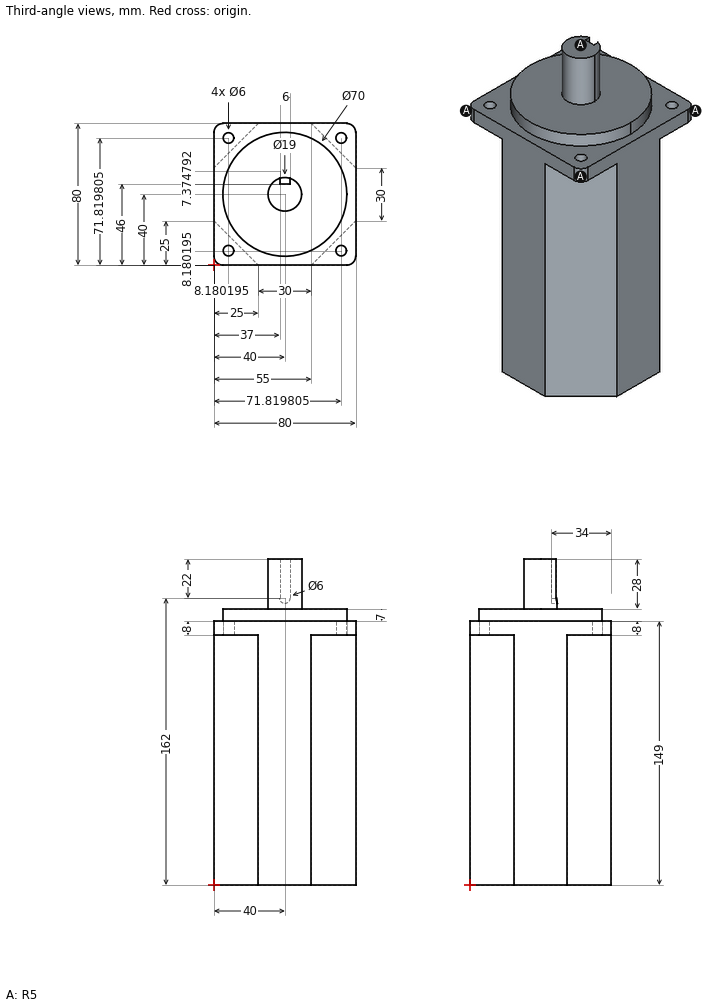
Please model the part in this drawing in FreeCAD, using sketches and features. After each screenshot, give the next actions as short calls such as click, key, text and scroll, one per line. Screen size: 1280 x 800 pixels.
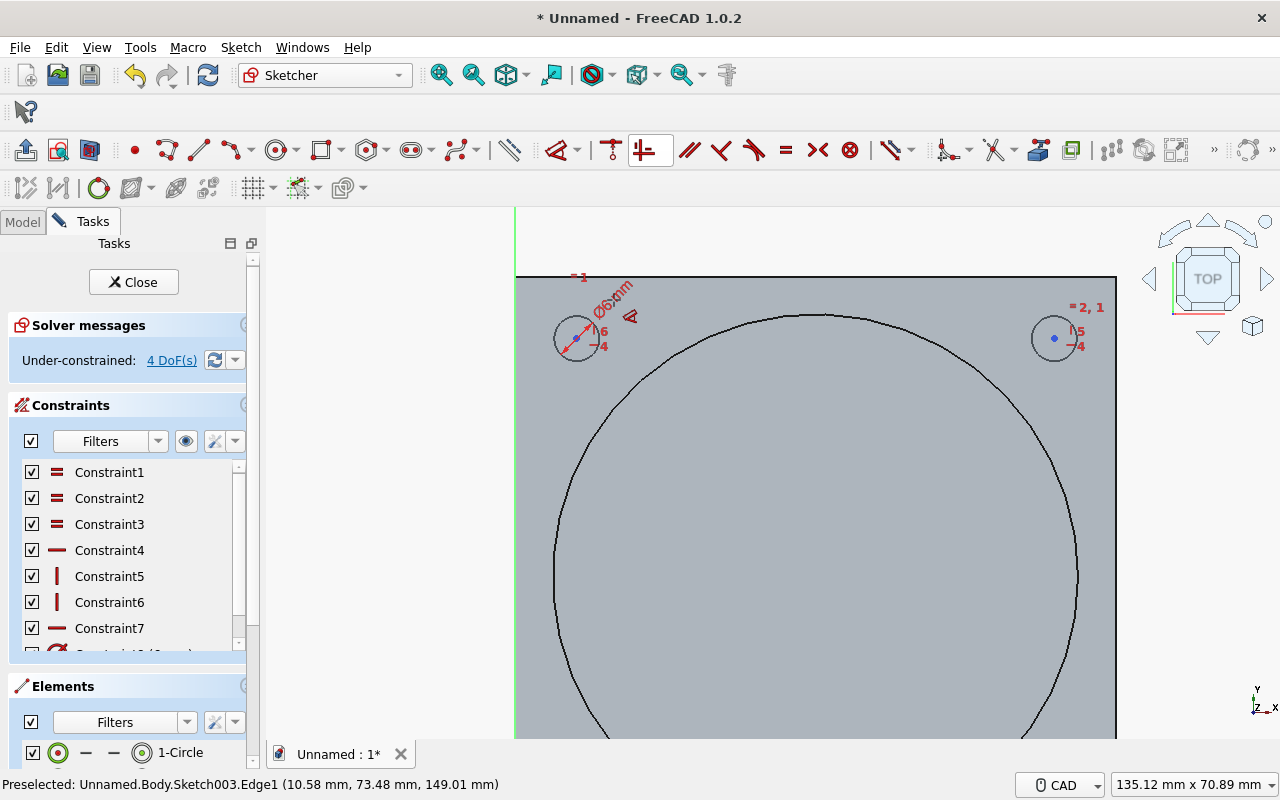
click(577, 339)
click(532, 305)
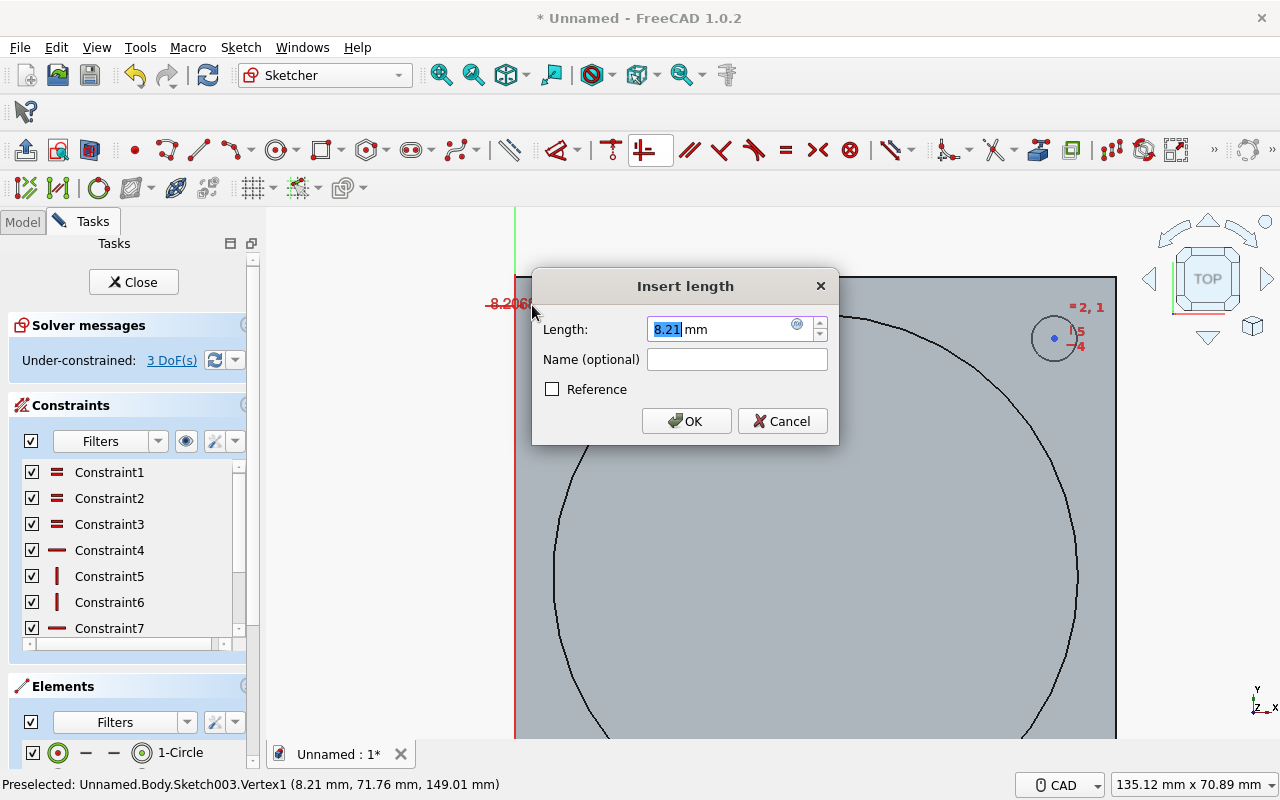
text(8.180195)
key(Return)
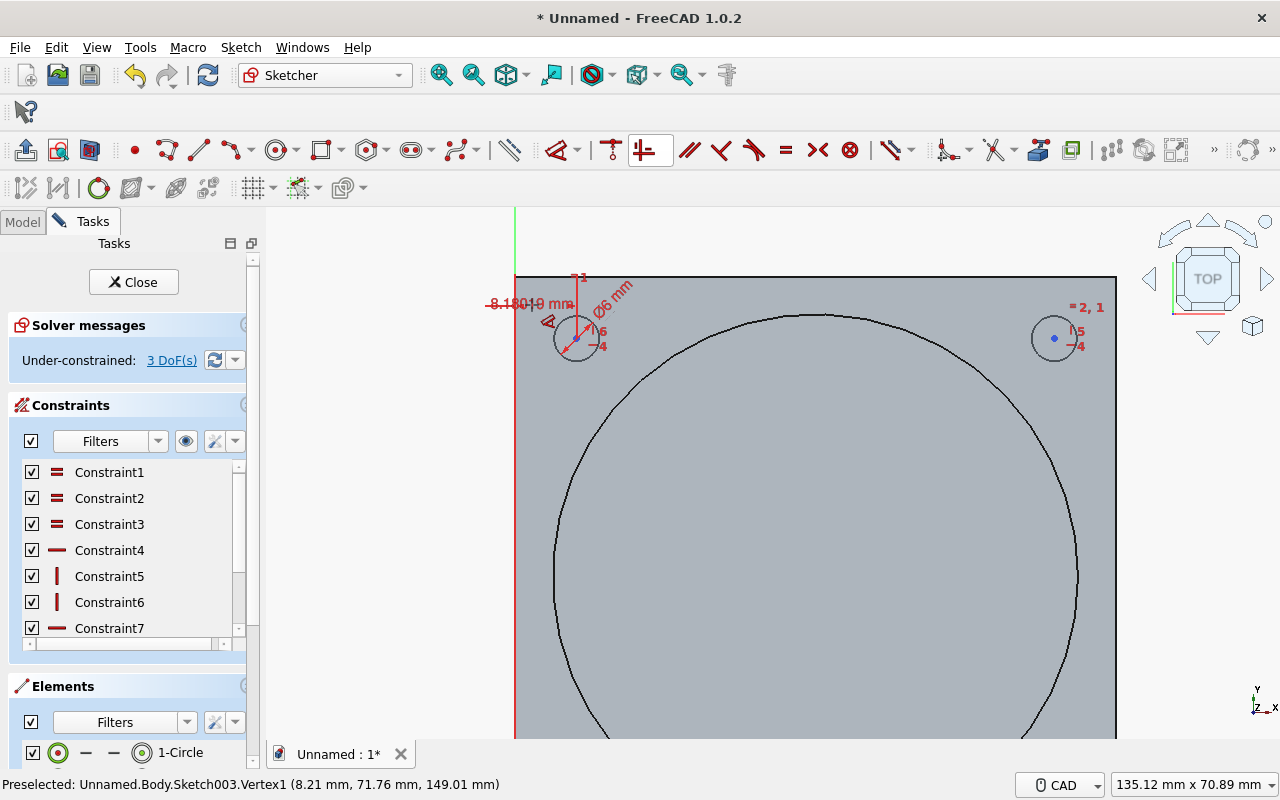
scroll(593, 323, down, 3)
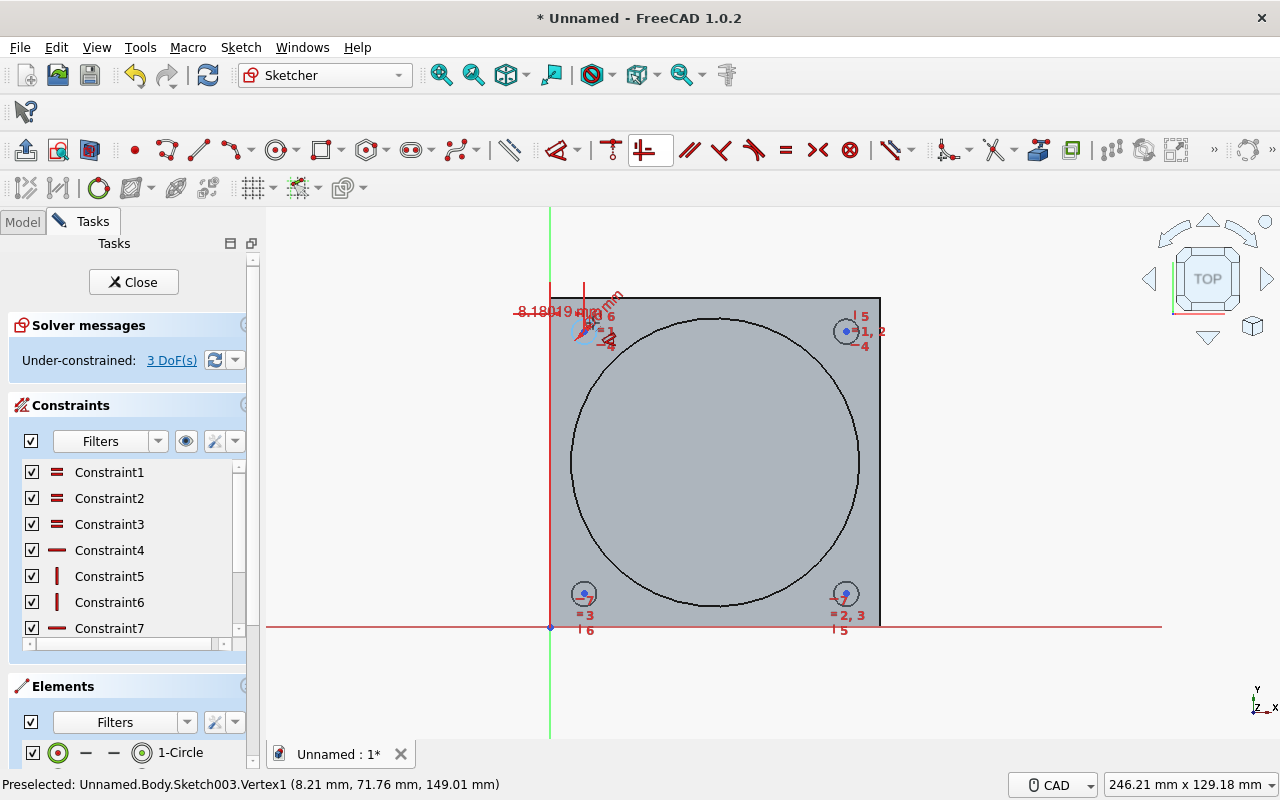
click(846, 594)
click(516, 611)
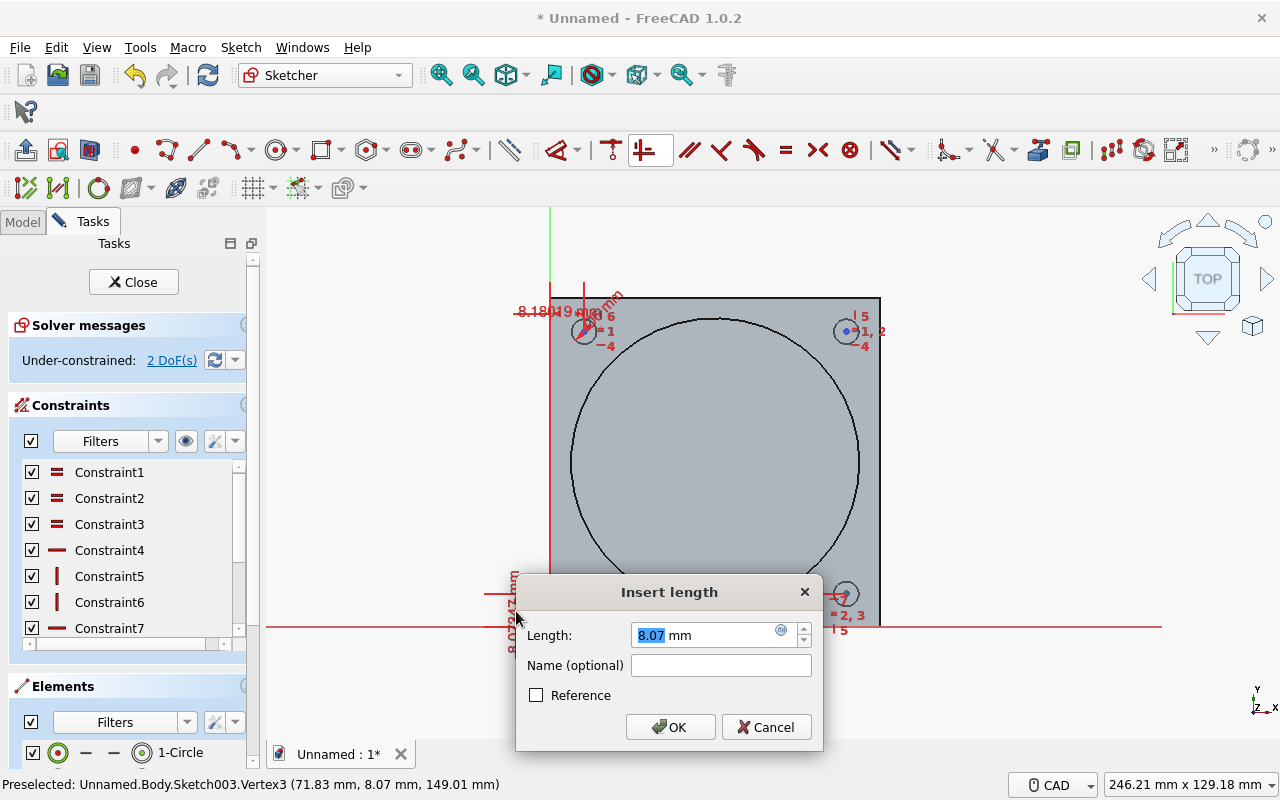
text(8.180195)
key(Return)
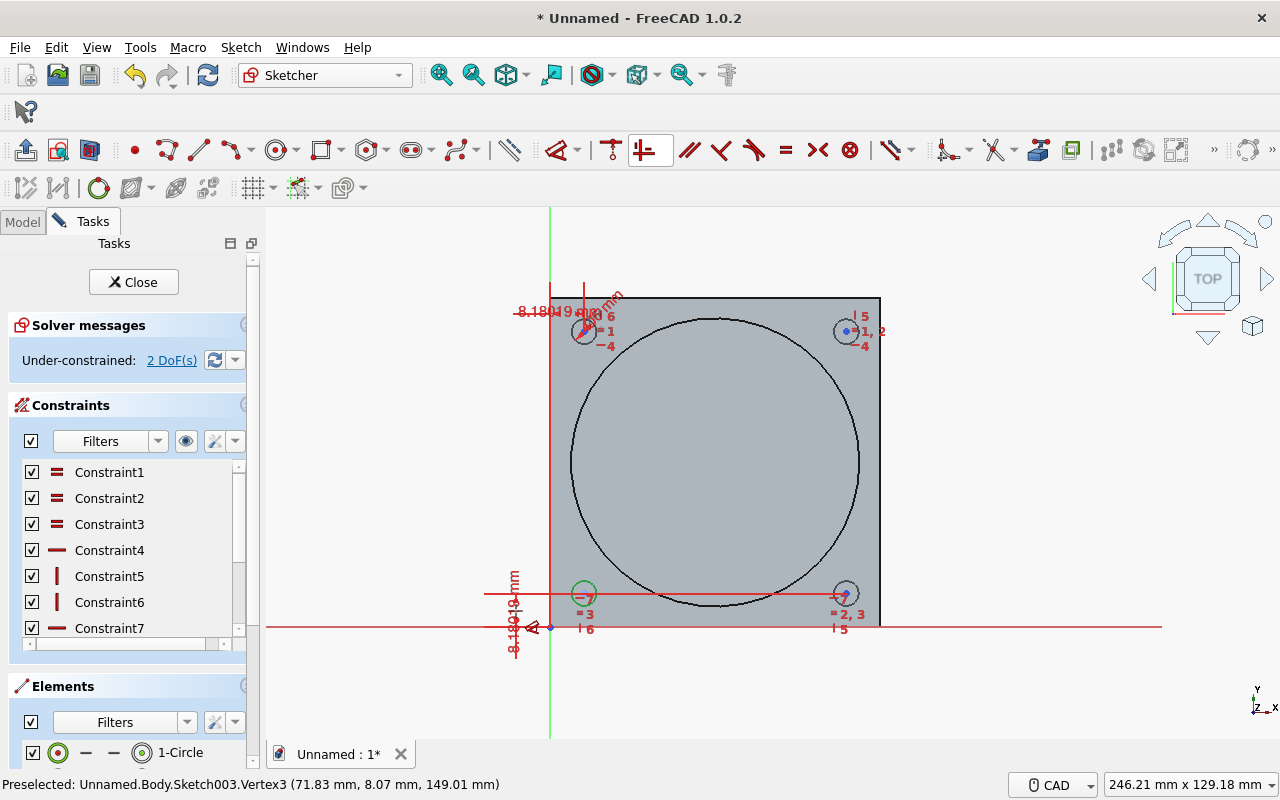
click(584, 332)
click(516, 479)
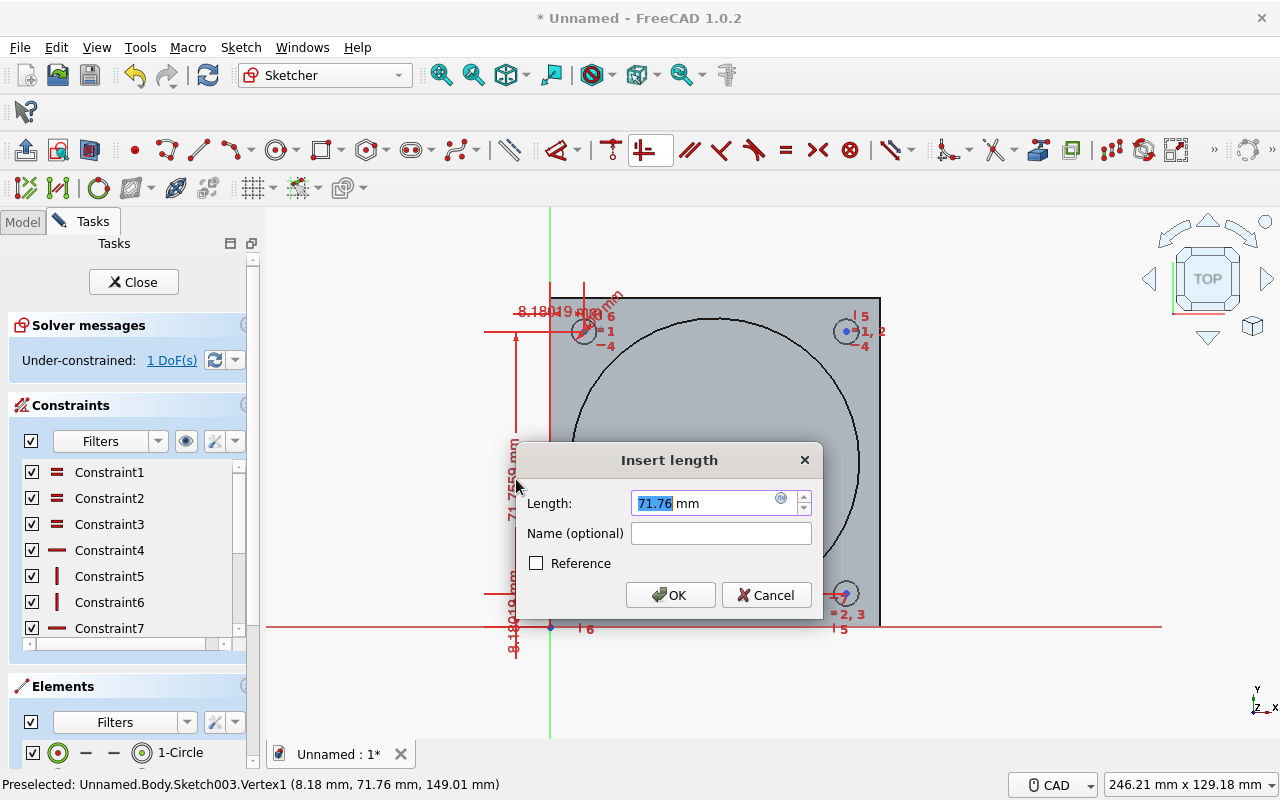
text(71.819805)
key(Return)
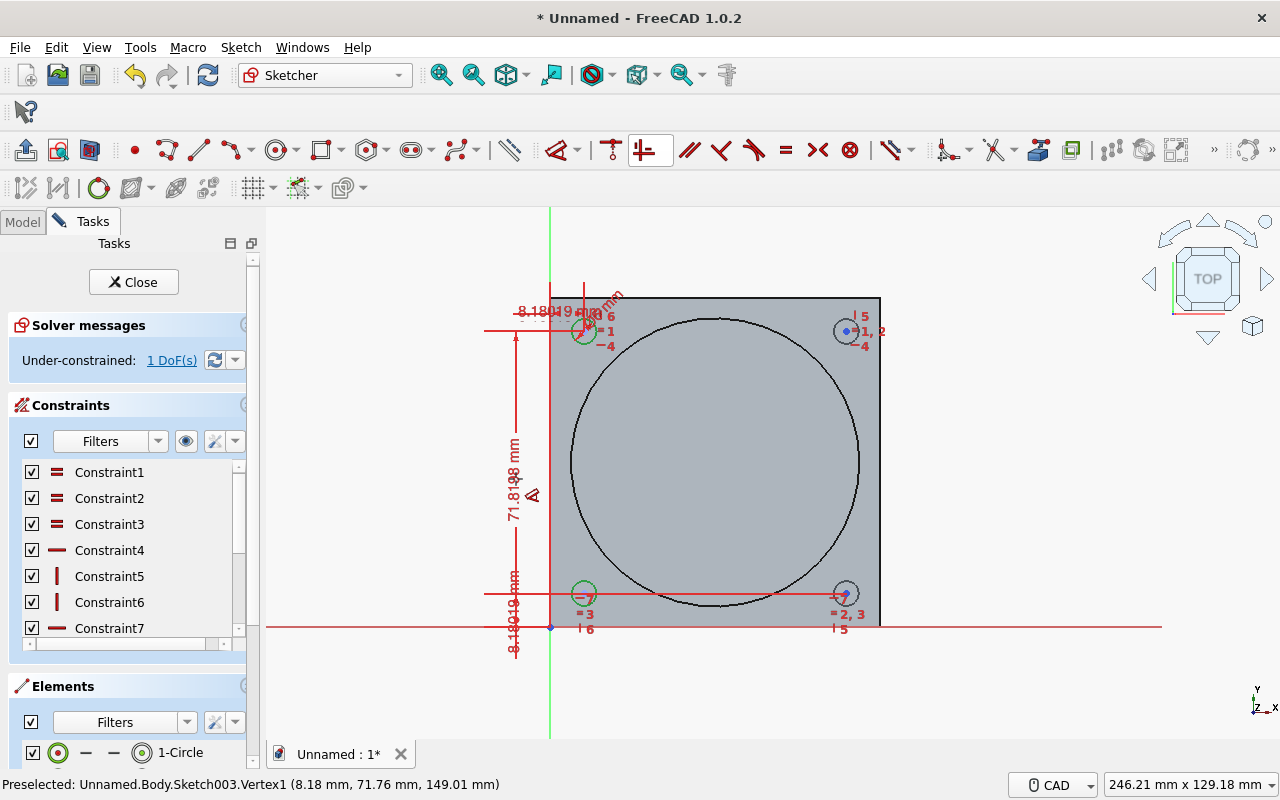
click(846, 331)
click(698, 661)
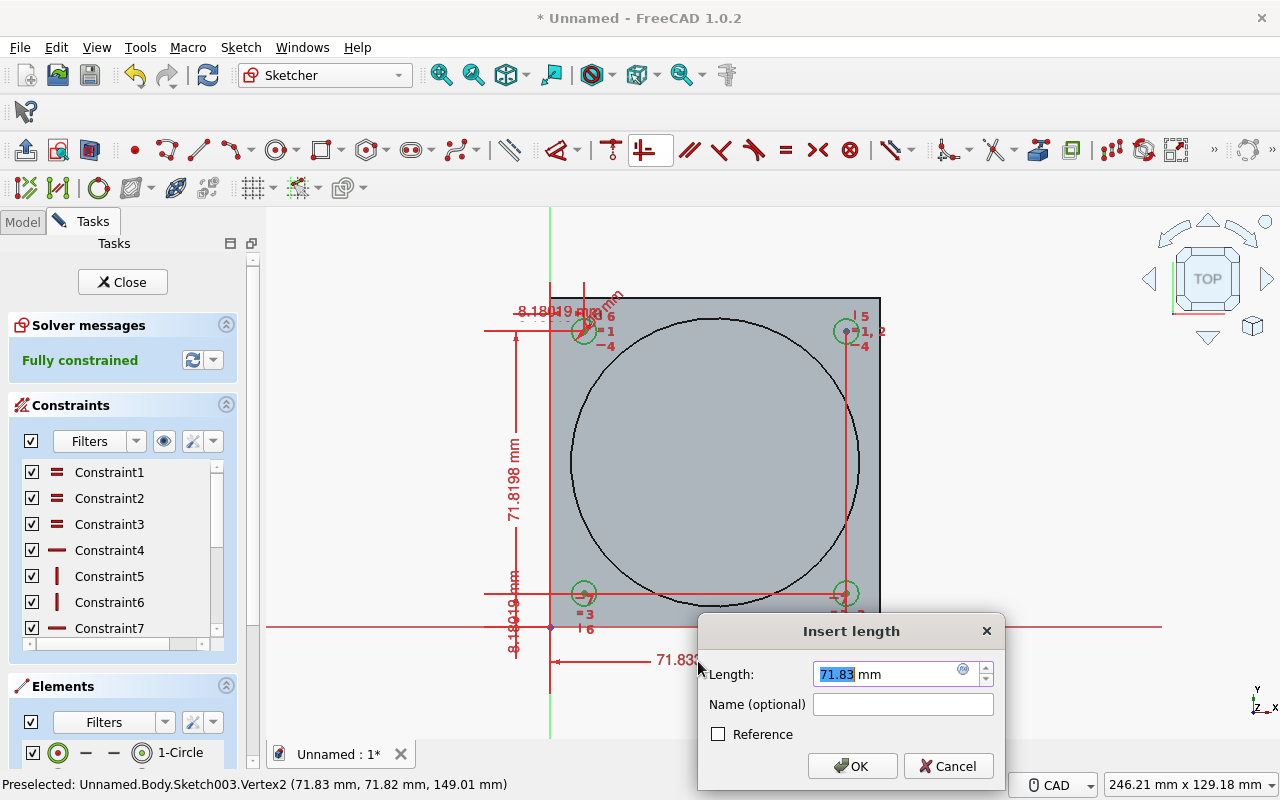
text(71.819805)
key(Return)
key(Escape)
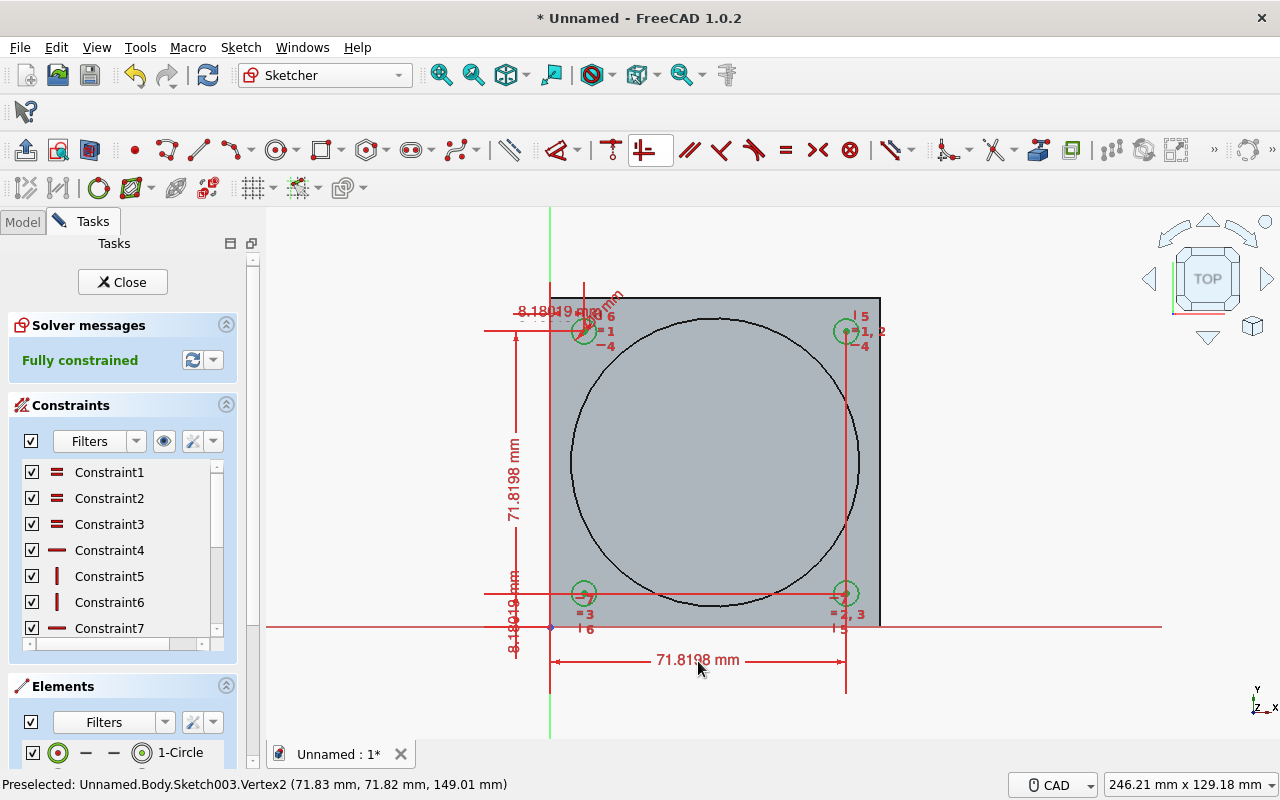
click(123, 282)